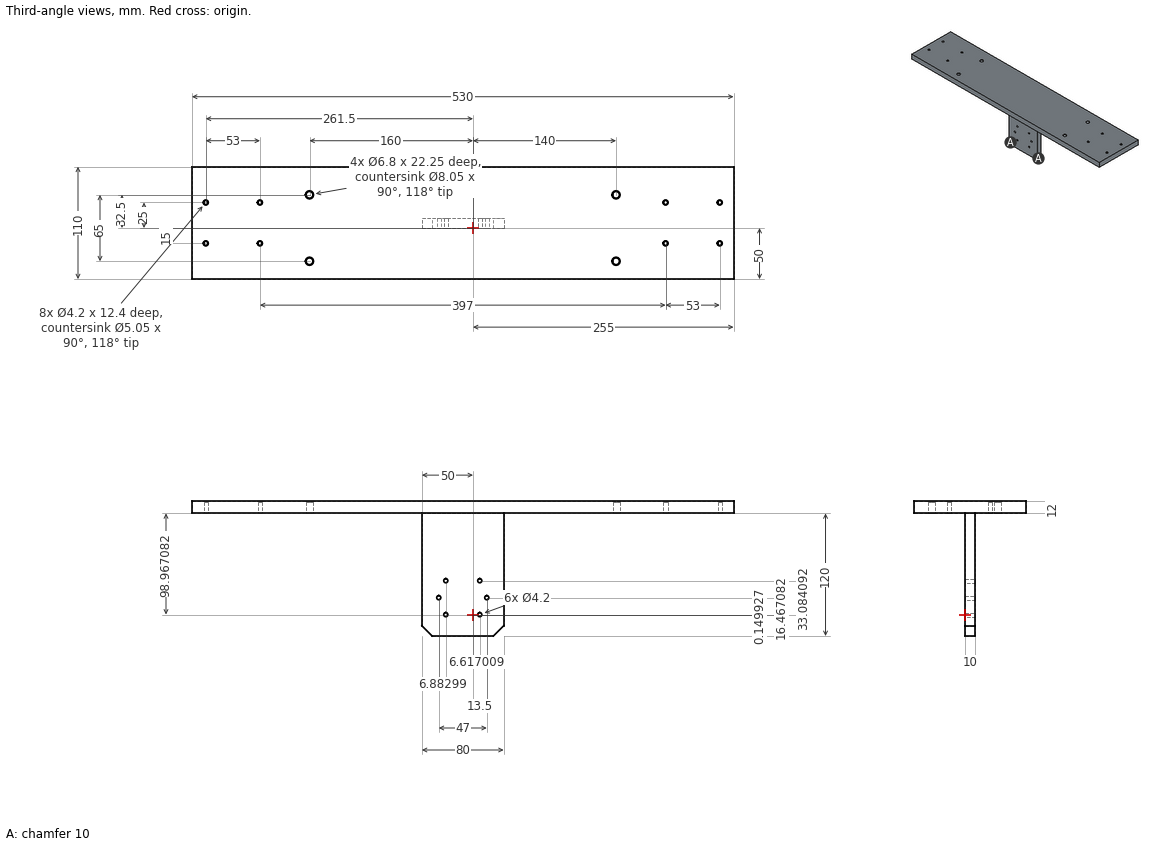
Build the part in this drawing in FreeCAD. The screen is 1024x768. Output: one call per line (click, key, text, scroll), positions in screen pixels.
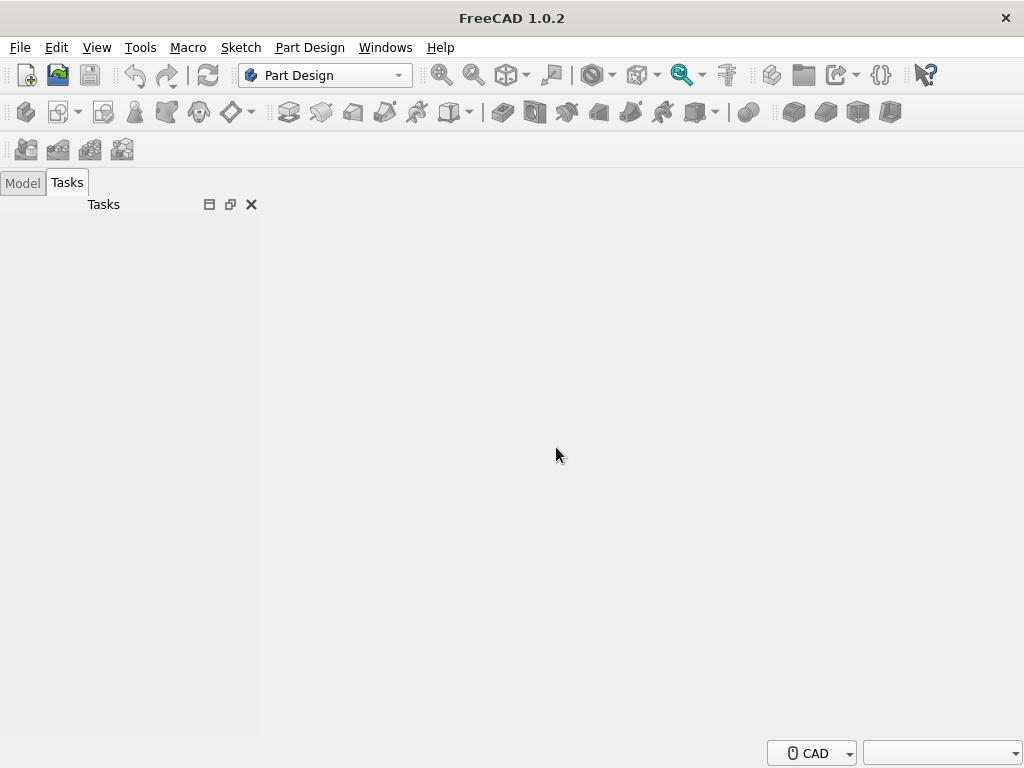
click(26, 76)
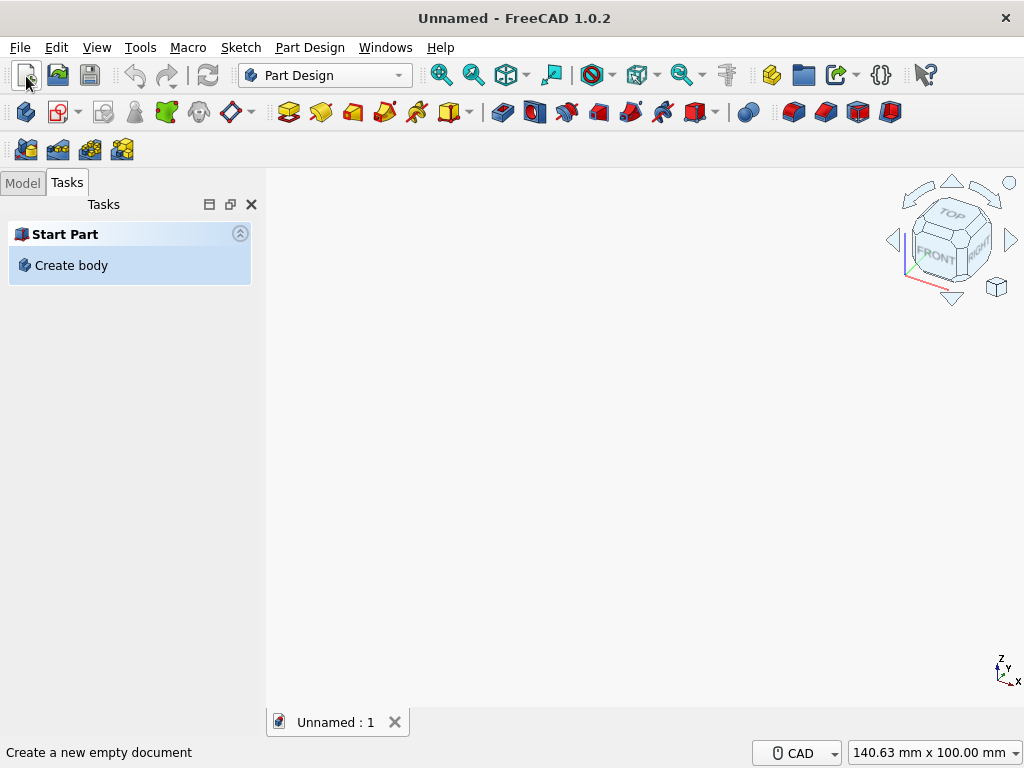
click(58, 112)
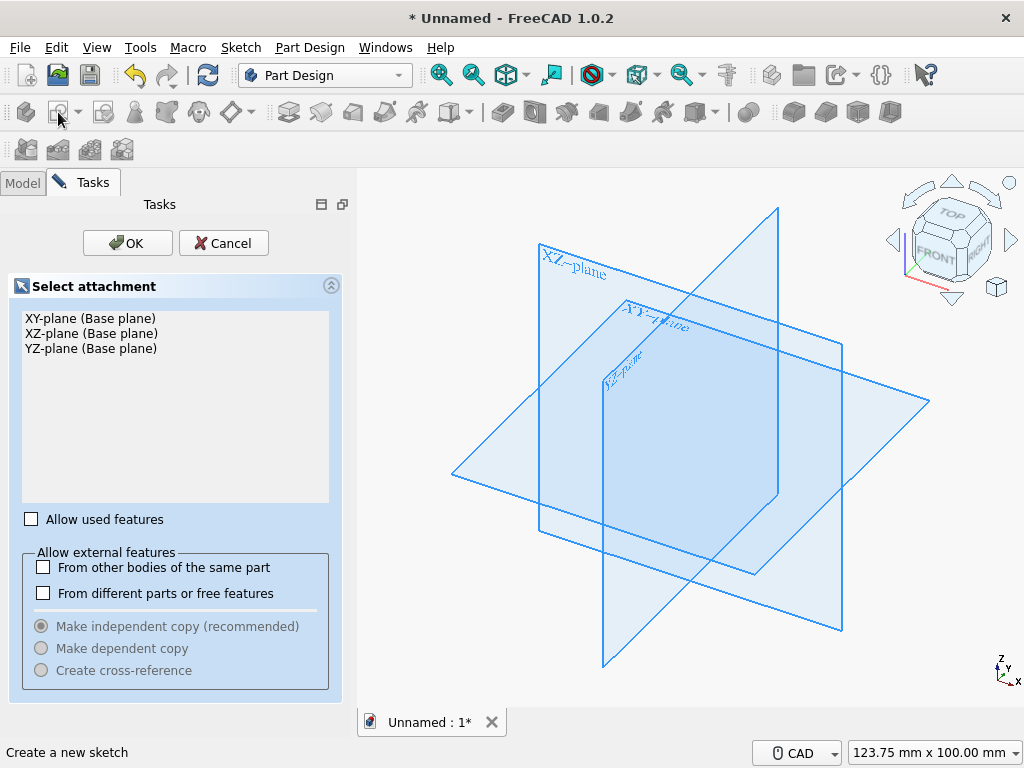
click(82, 334)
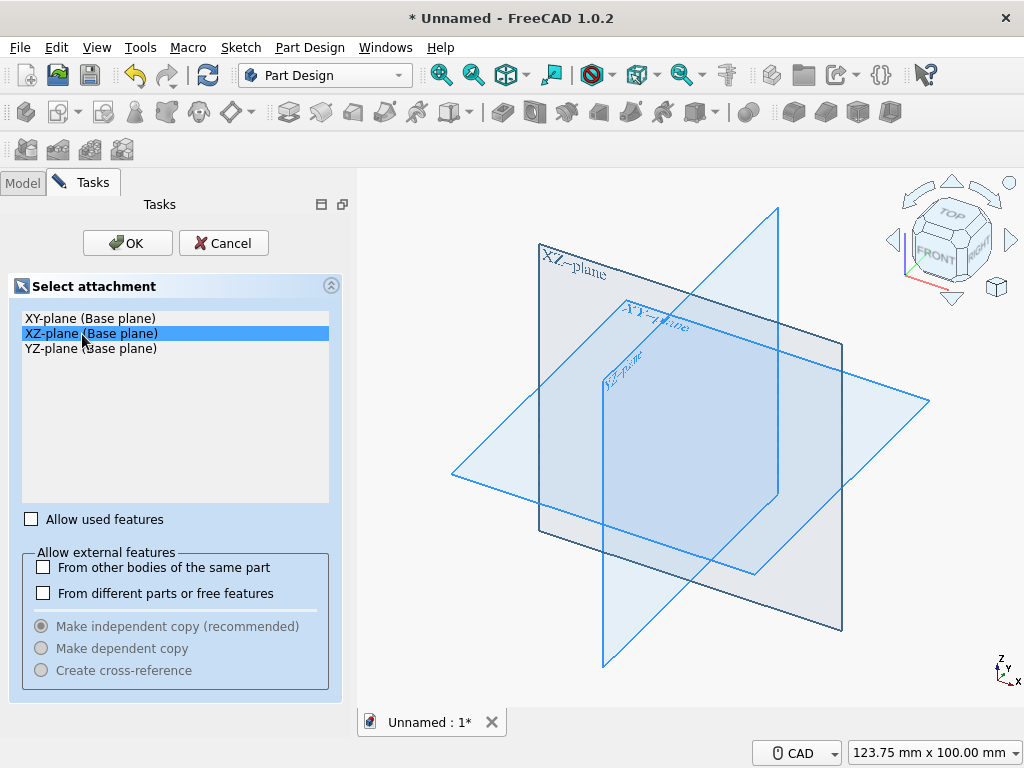
click(128, 243)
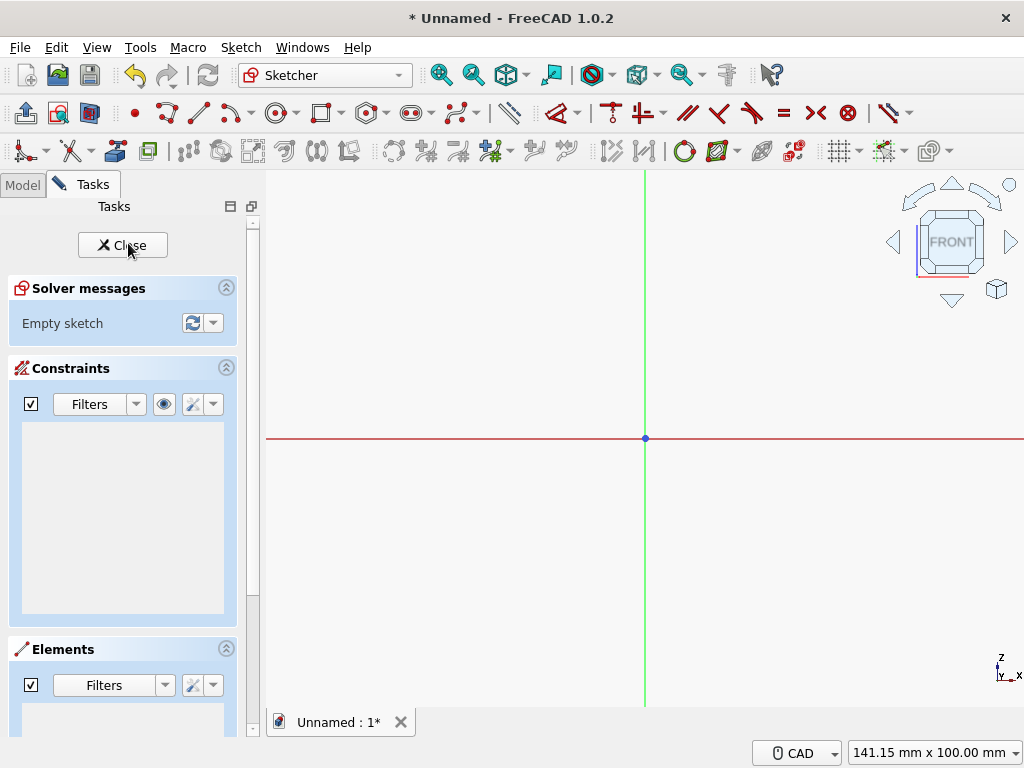
scroll(558, 679, down, 3)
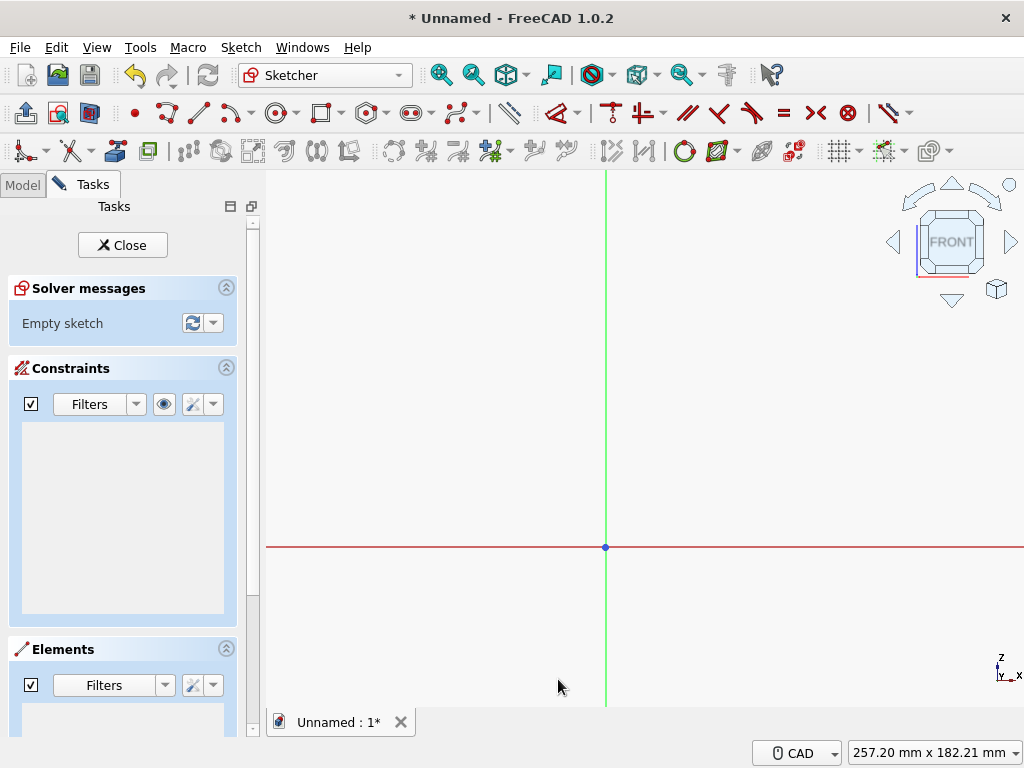
key(g)
key(r)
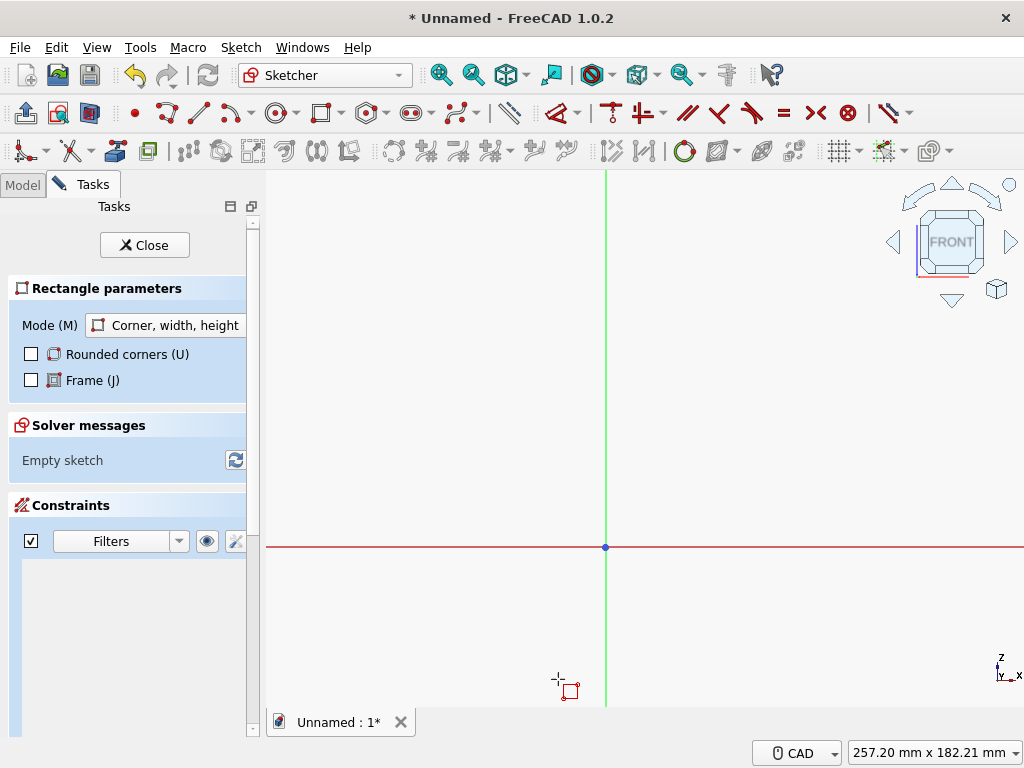
click(459, 256)
move(694, 609)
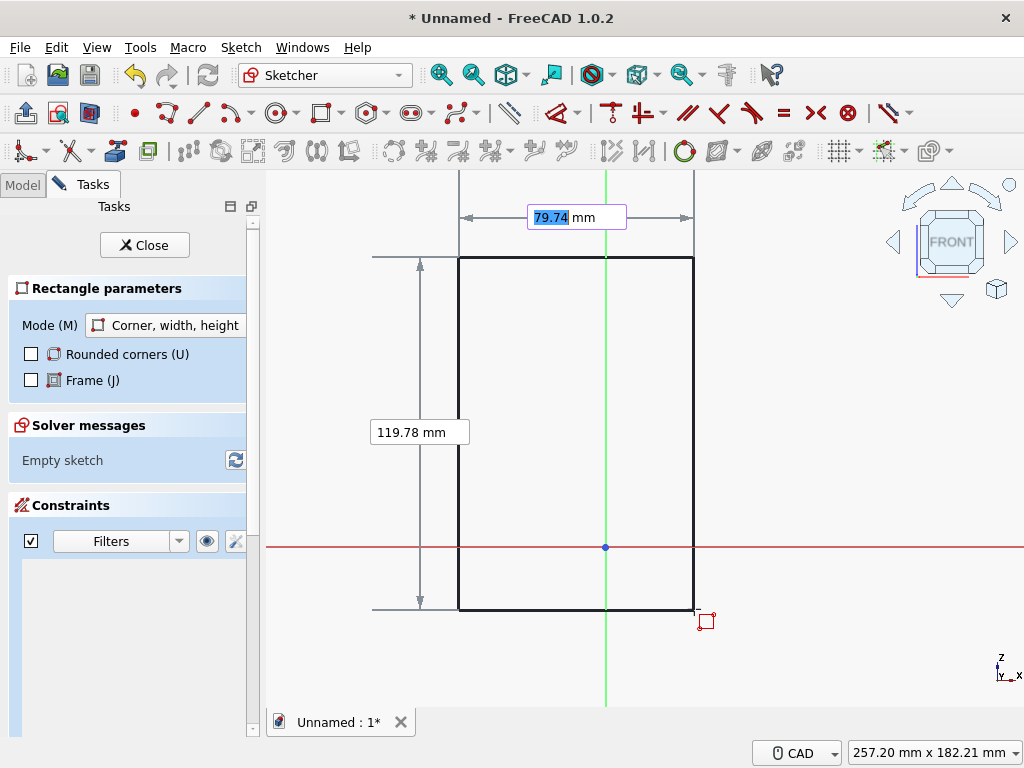
text(80)
key(Tab)
text(120)
key(Return)
key(Escape)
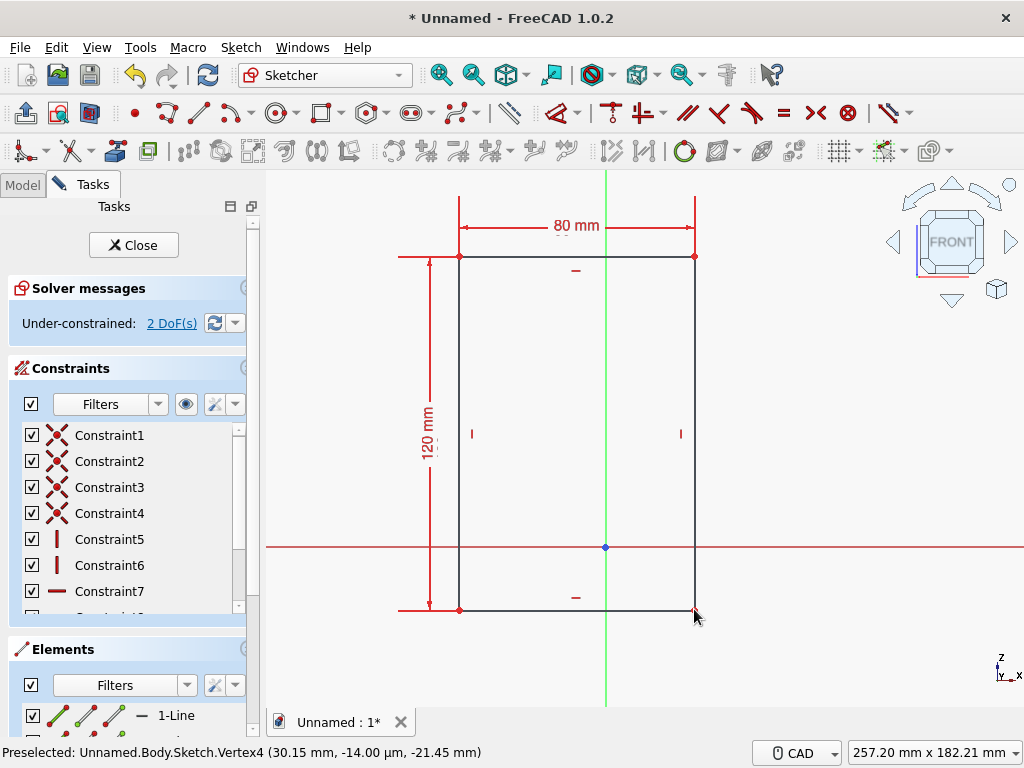
click(459, 257)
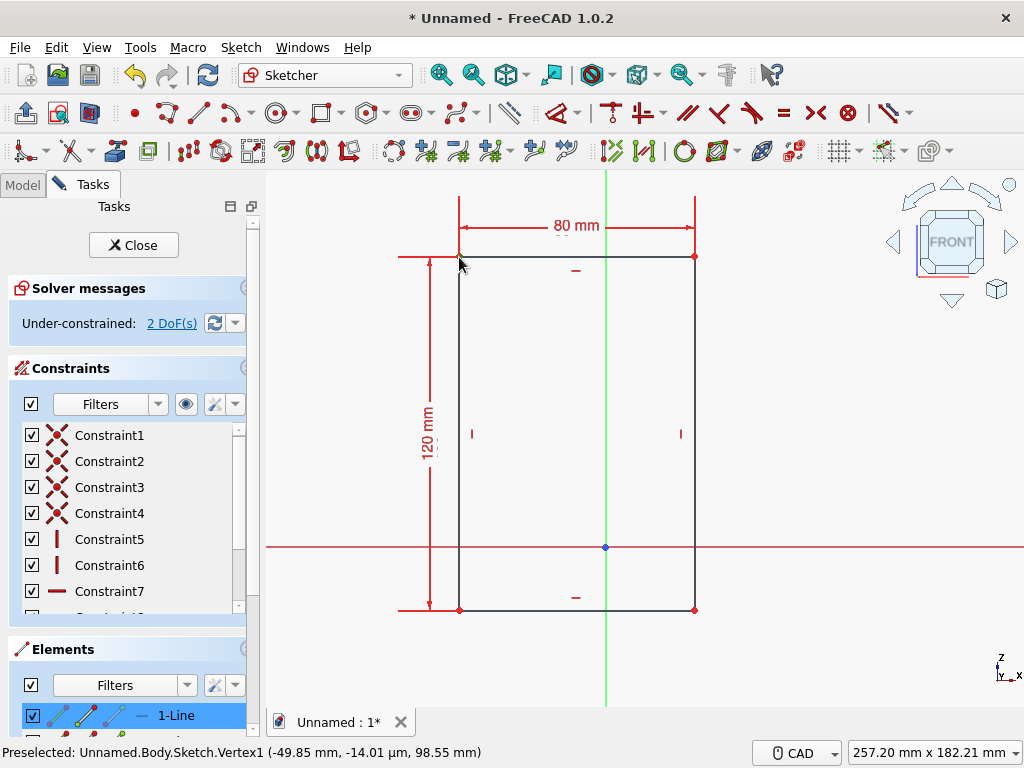
key(l)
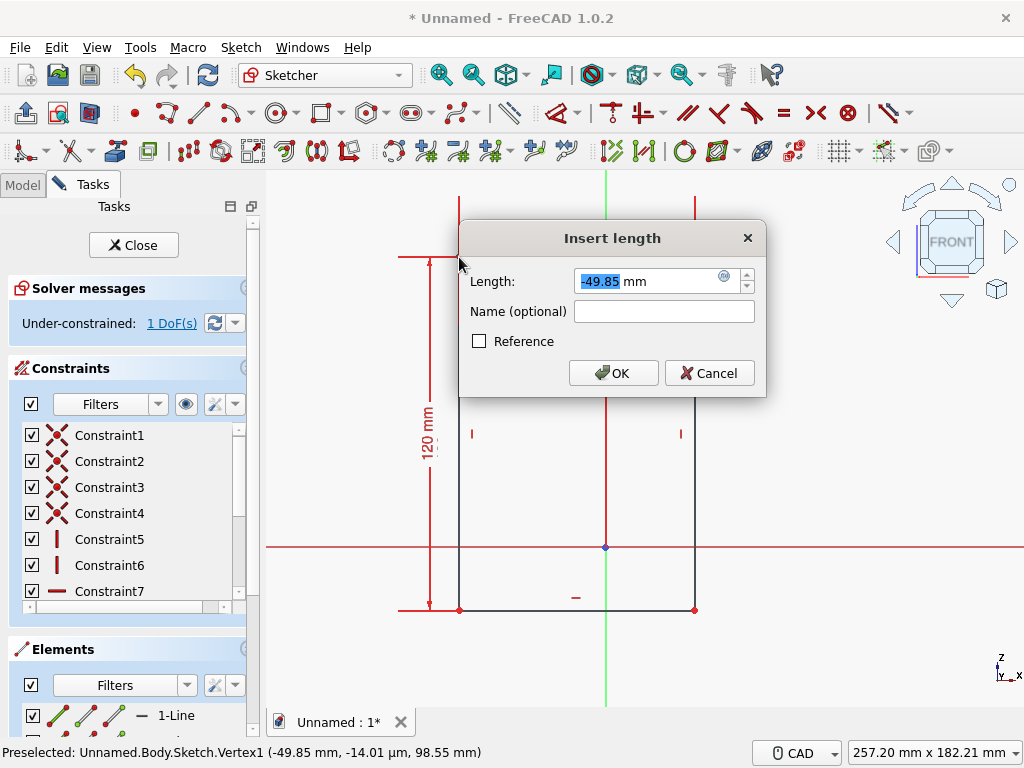
text(-50)
key(Return)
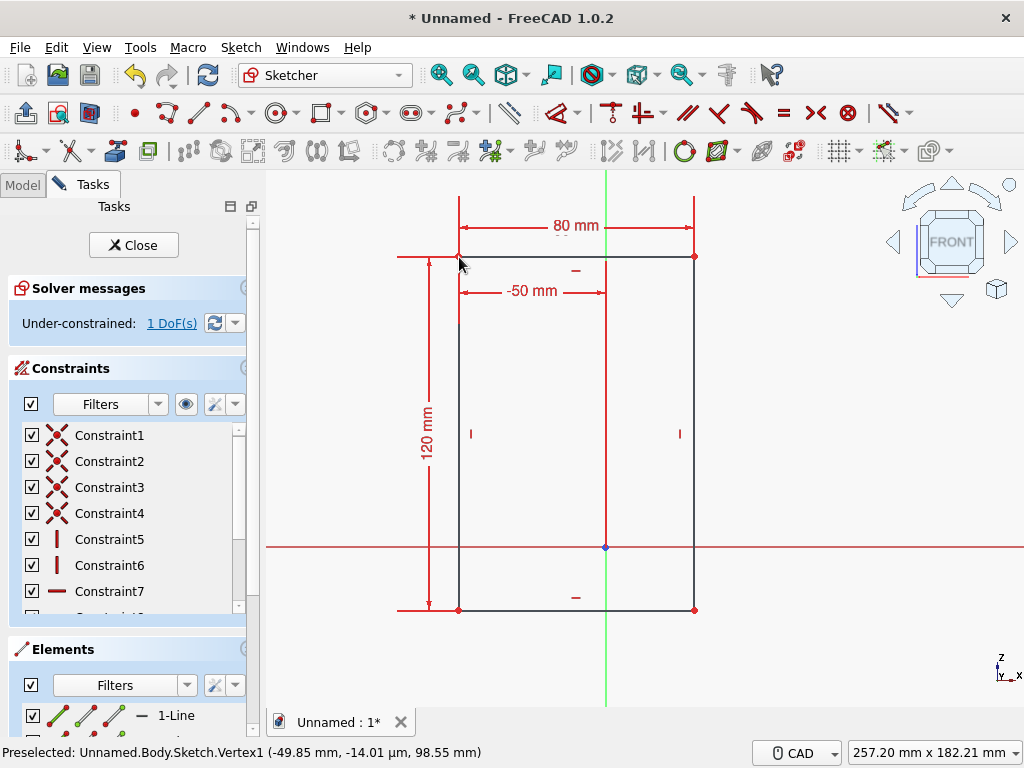
click(459, 257)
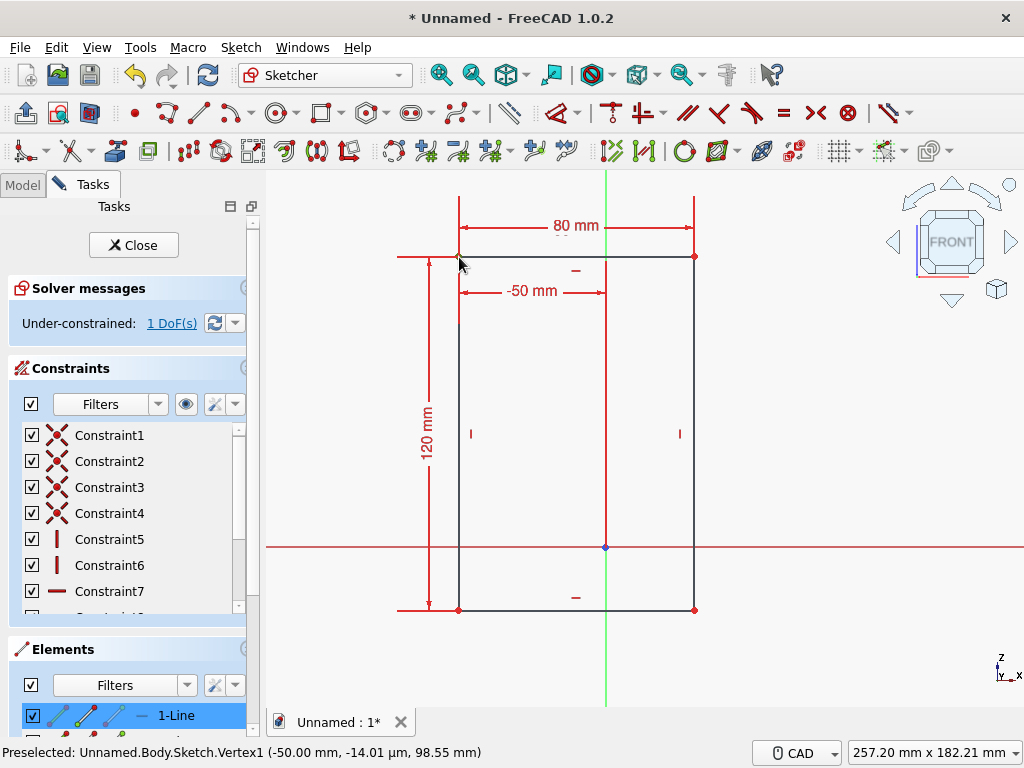
key(i)